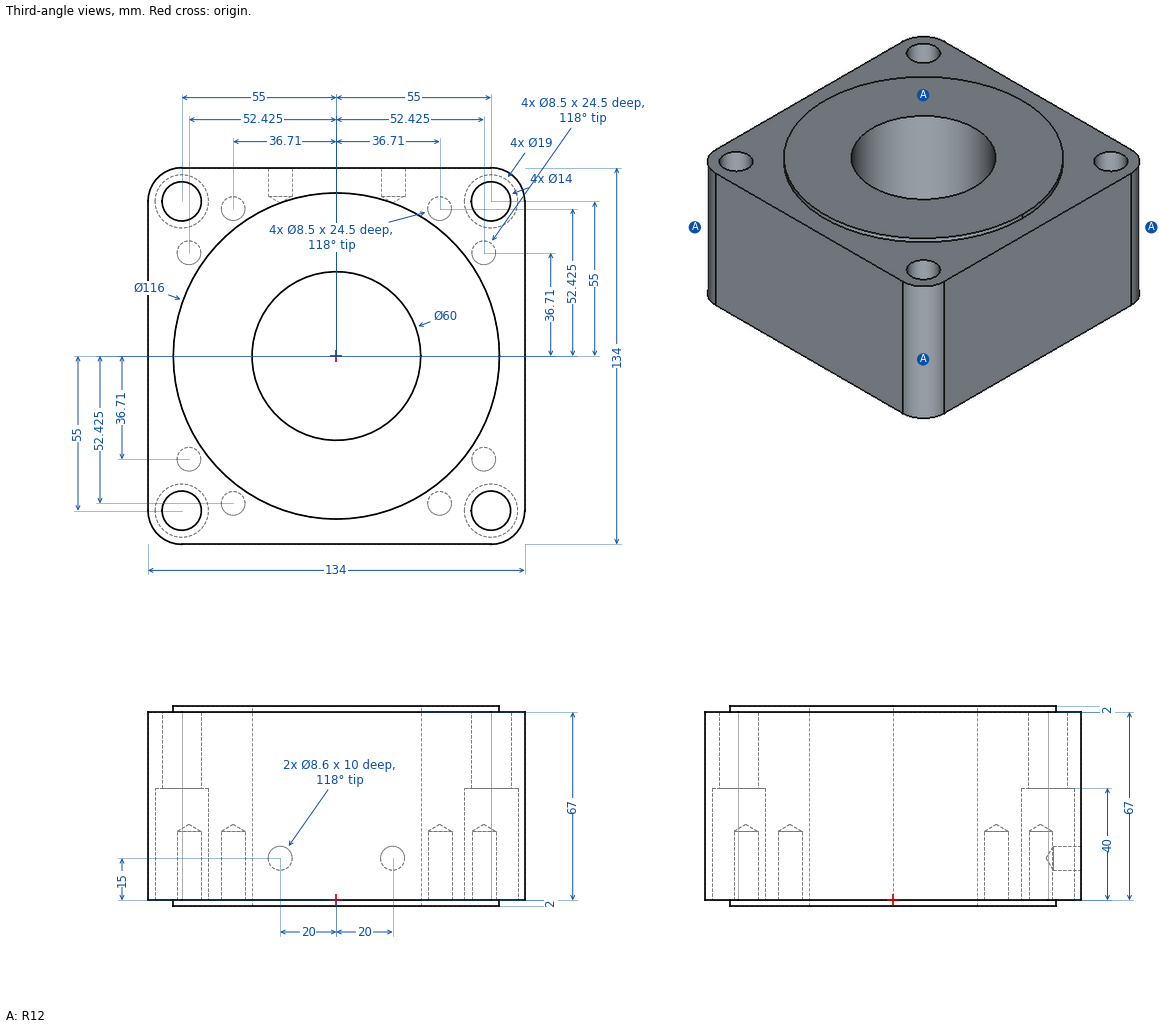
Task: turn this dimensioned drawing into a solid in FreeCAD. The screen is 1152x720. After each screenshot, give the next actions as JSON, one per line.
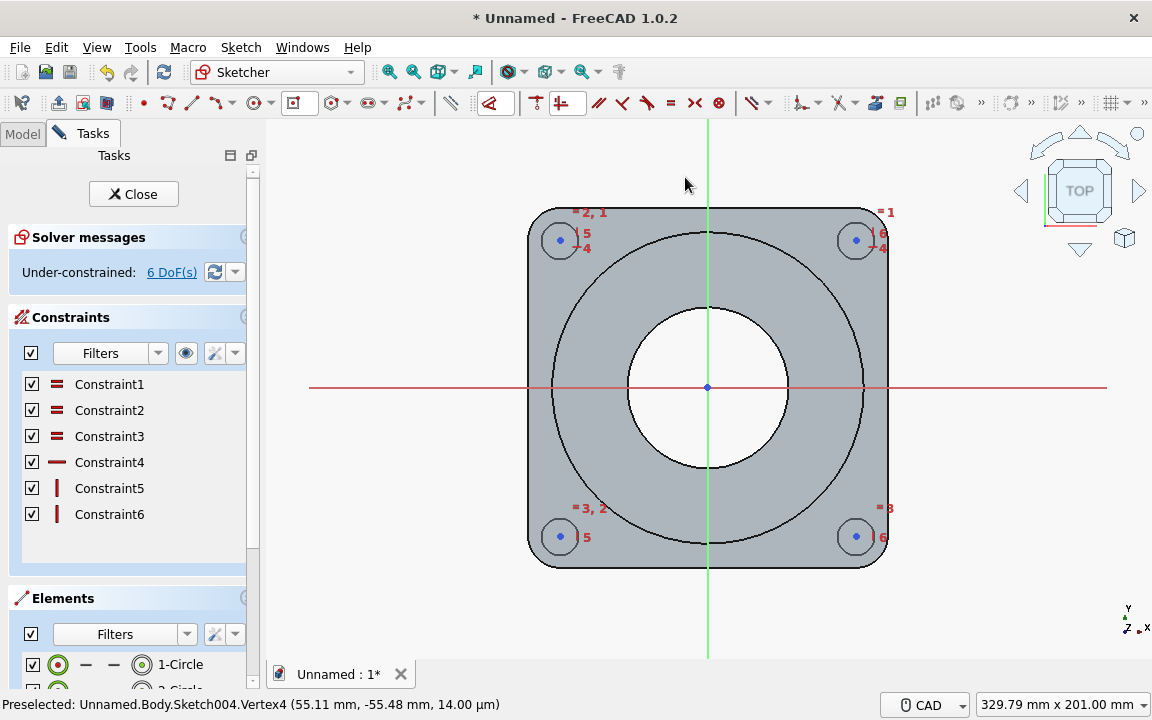
{"action": "left_click", "coordinate": [560, 537]}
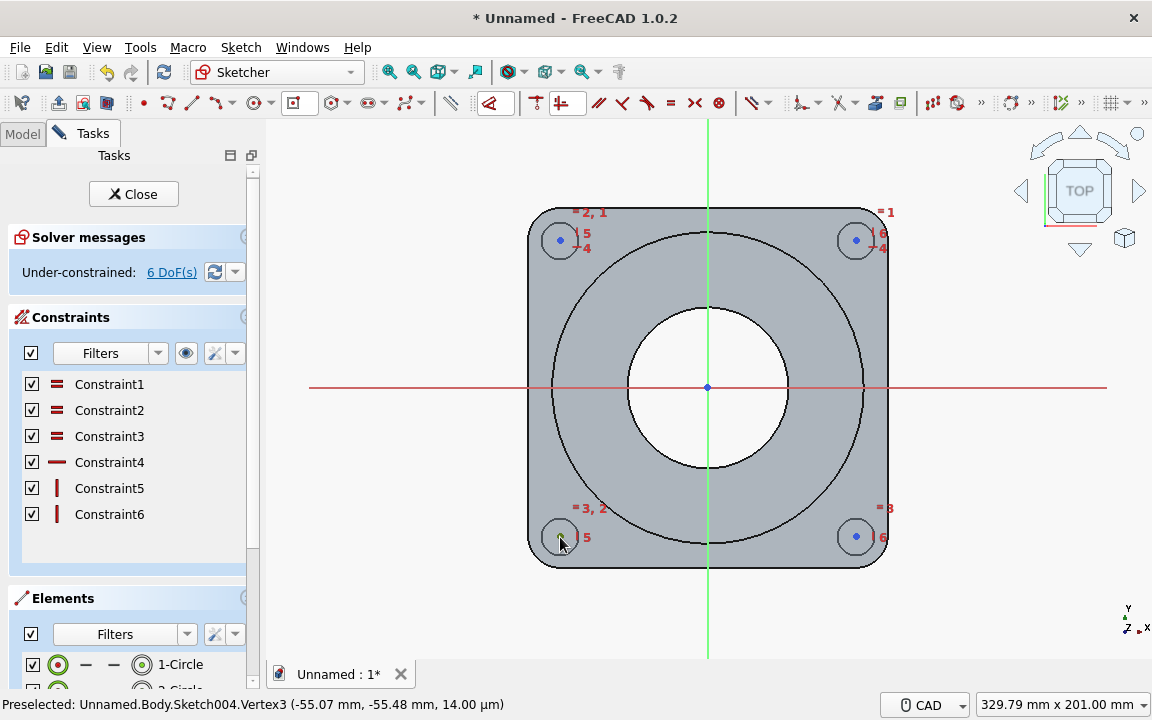
{"action": "left_click", "coordinate": [856, 537]}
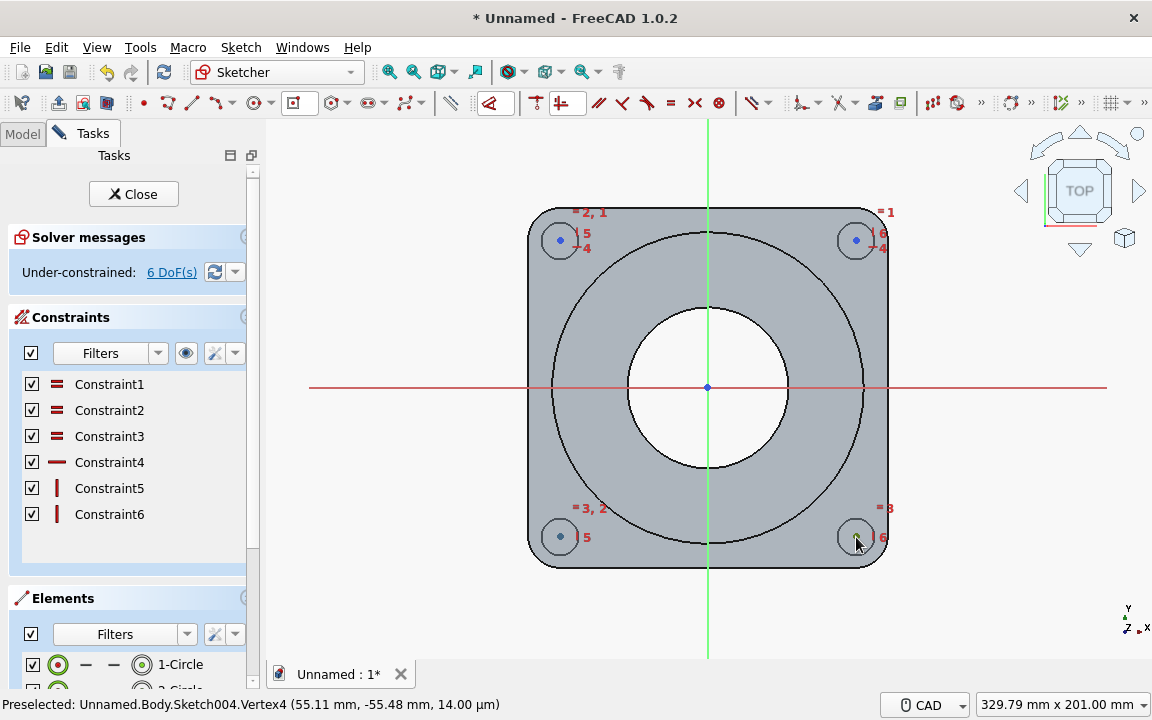
{"action": "left_click", "coordinate": [580, 104]}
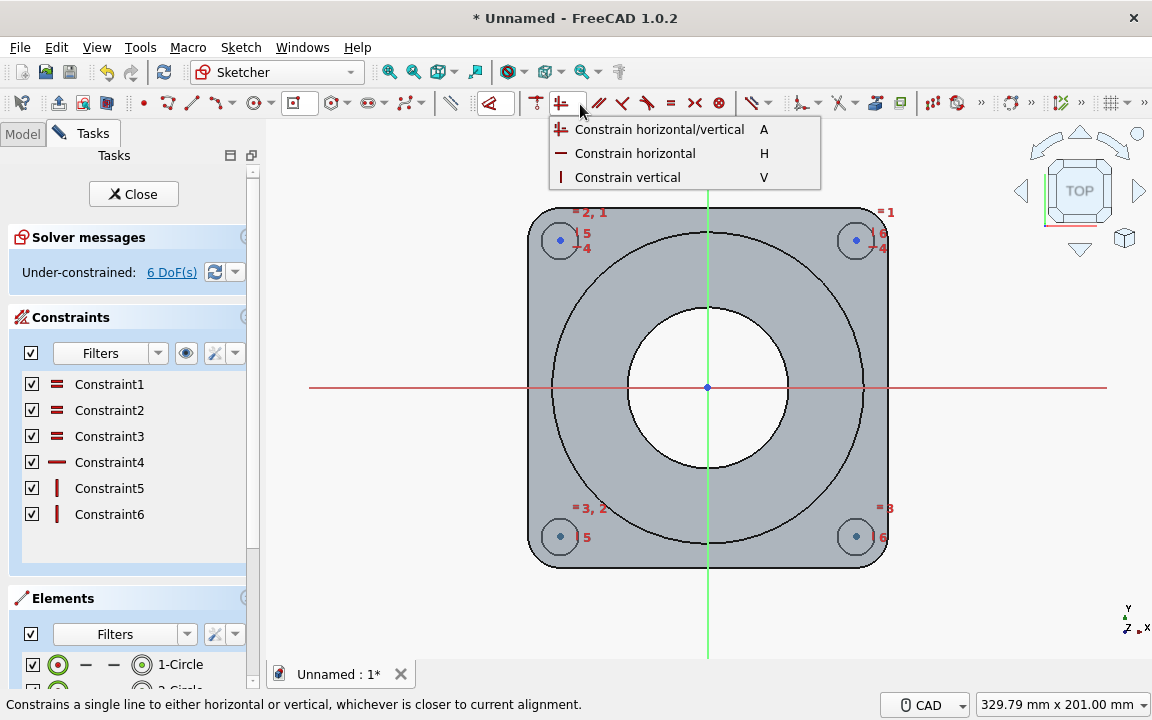
{"action": "left_click", "coordinate": [685, 153]}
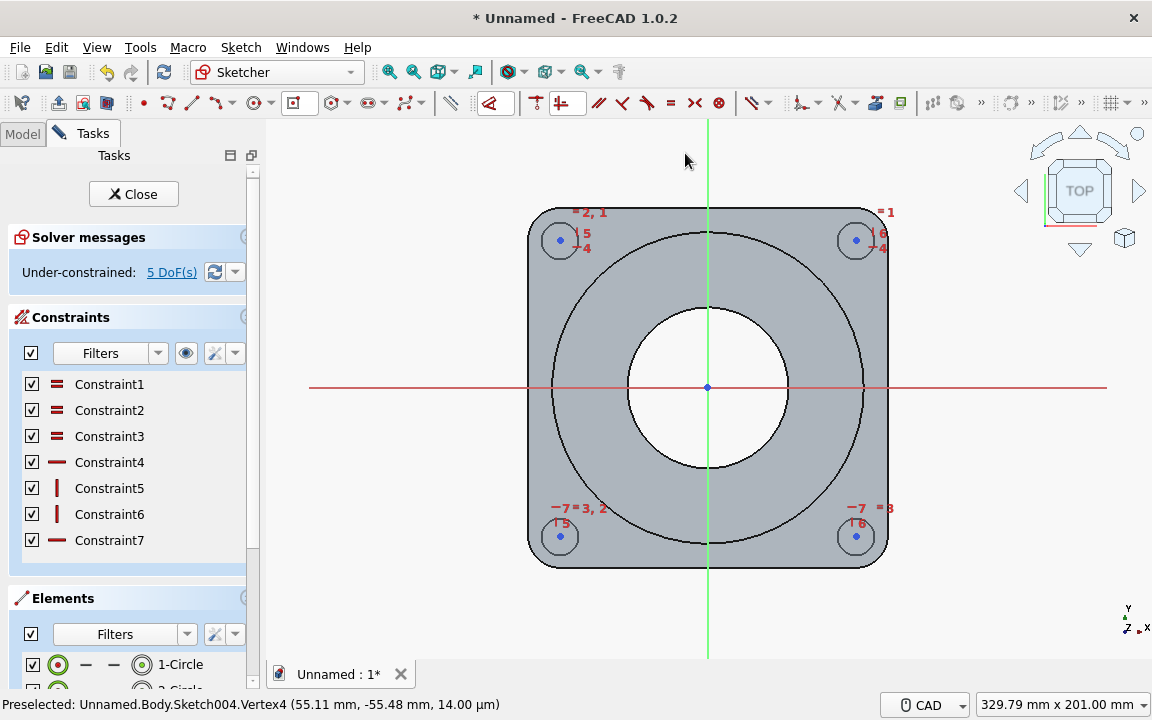
{"action": "left_click", "coordinate": [843, 228]}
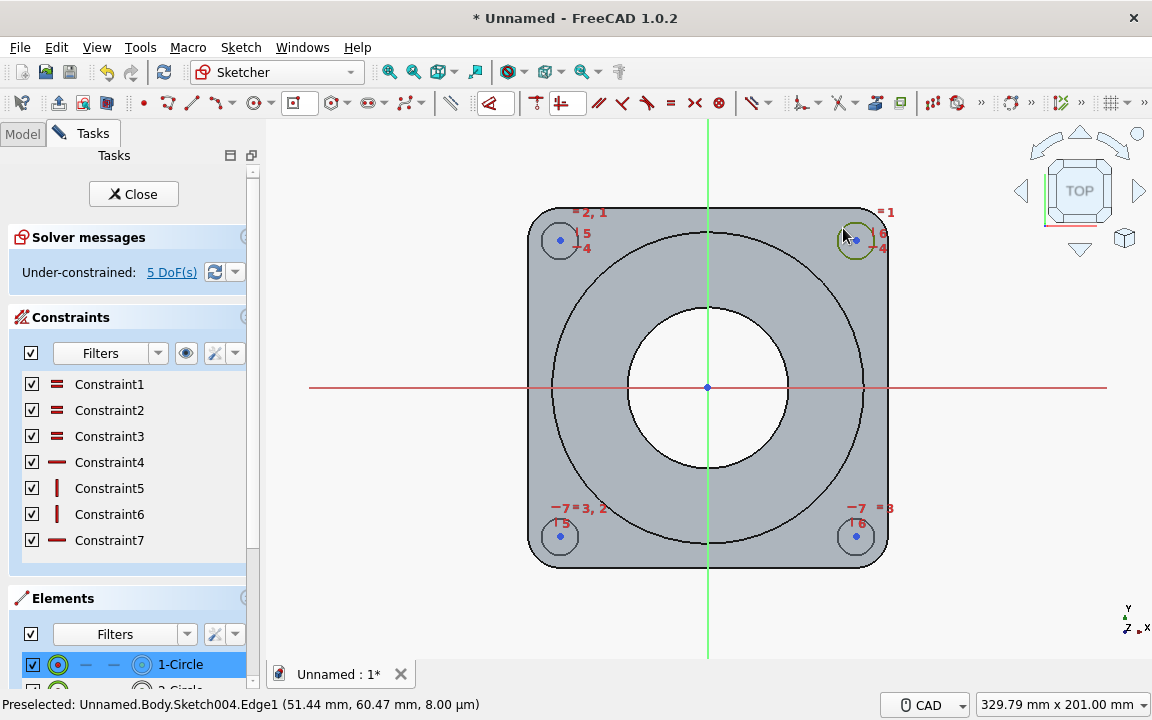
{"action": "key", "text": "k o"}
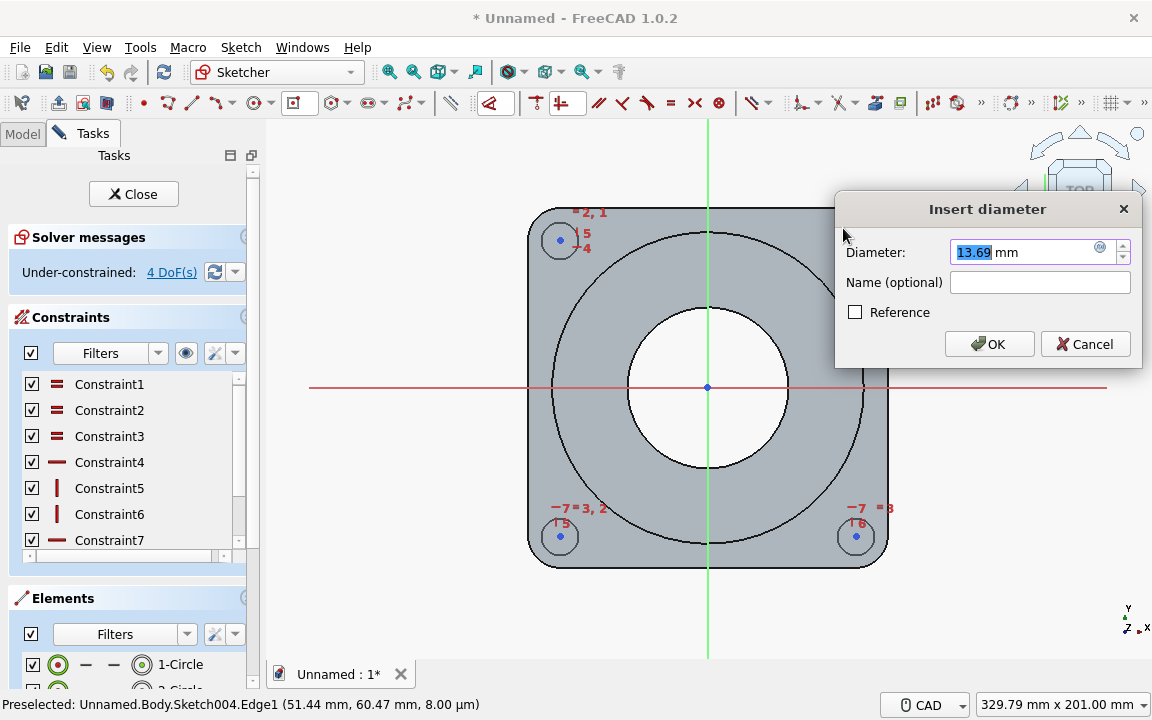
{"action": "type", "text": "14"}
{"action": "key", "text": "Return"}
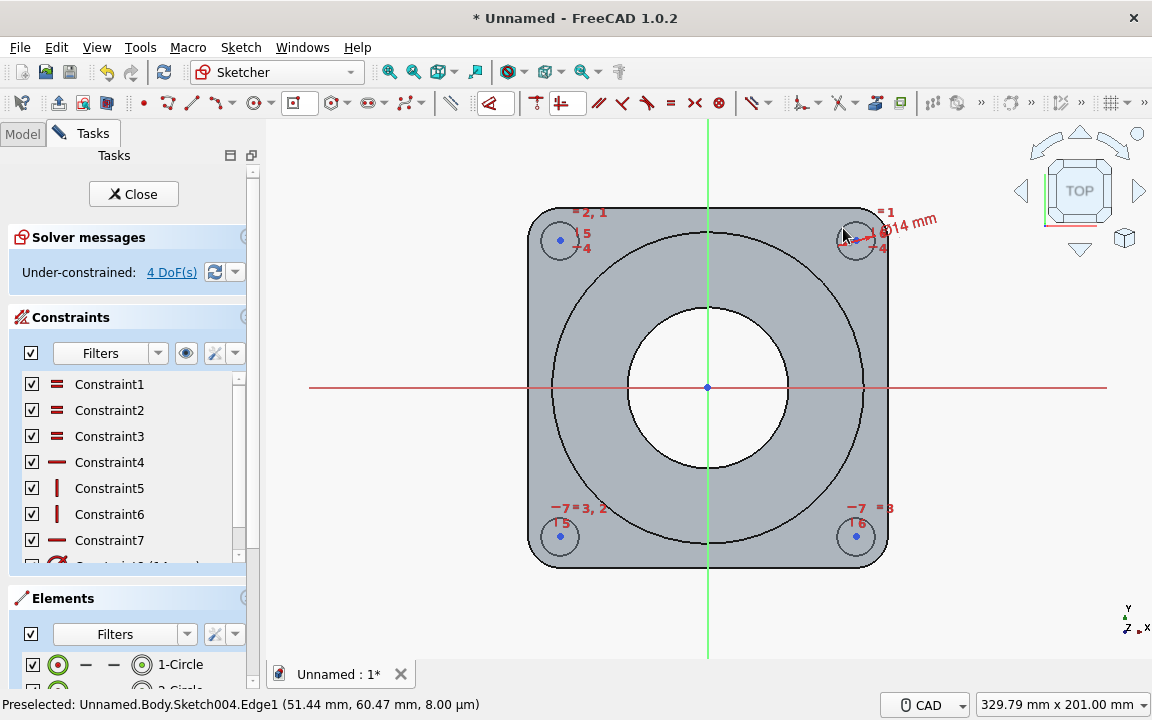
{"action": "left_click", "coordinate": [856, 241]}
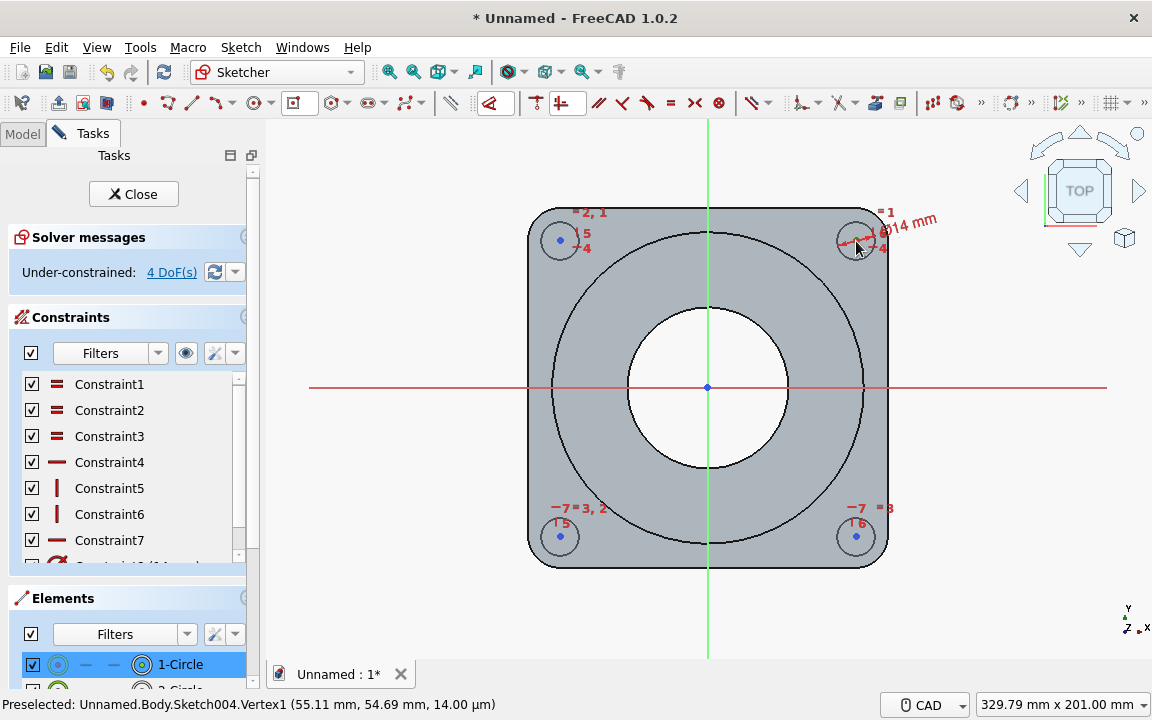
{"action": "left_click", "coordinate": [508, 104]}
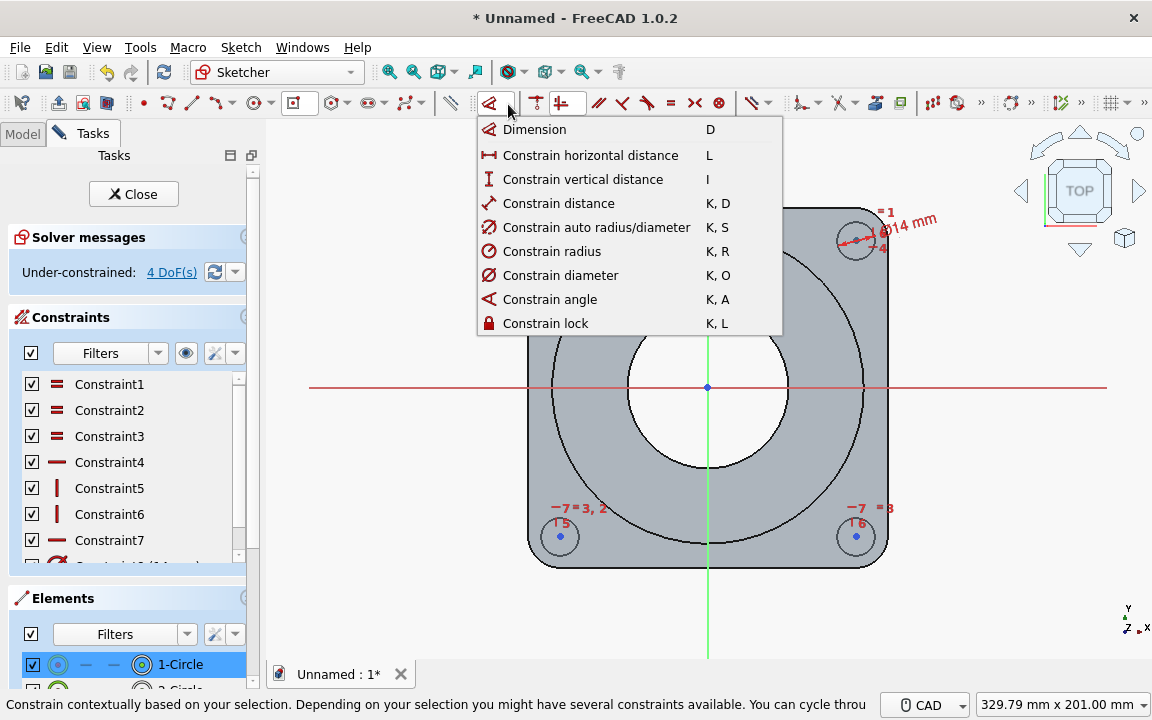
{"action": "left_click", "coordinate": [630, 155]}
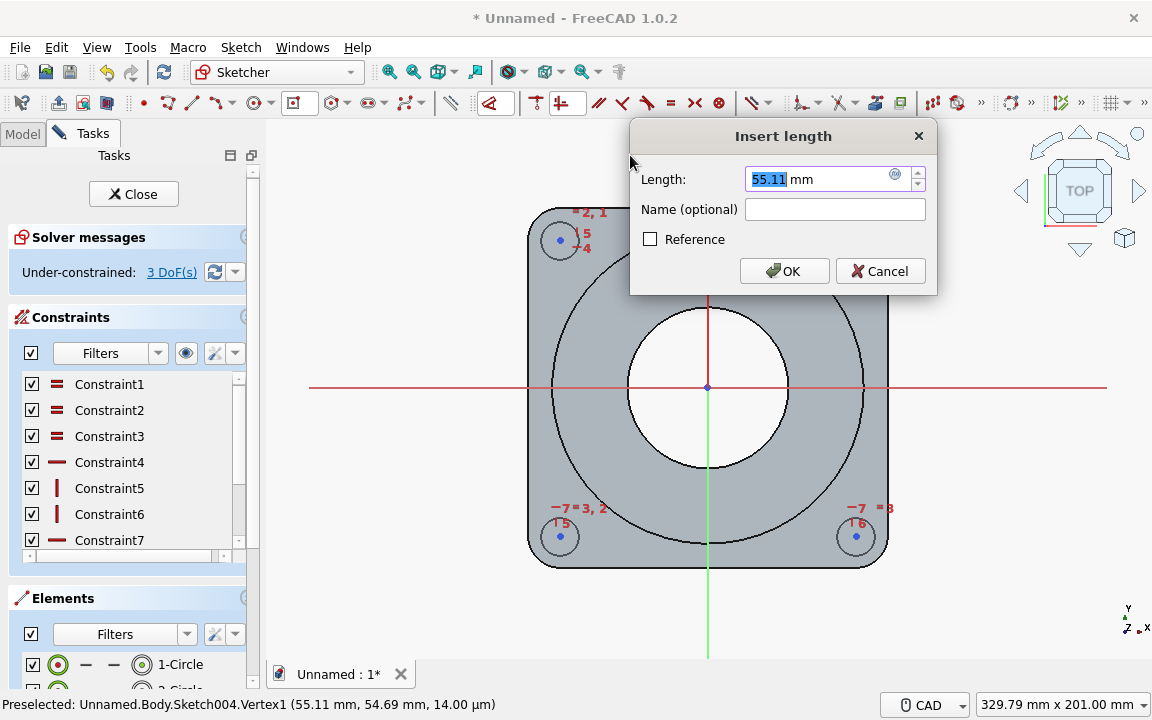
{"action": "type", "text": "55"}
{"action": "key", "text": "Return"}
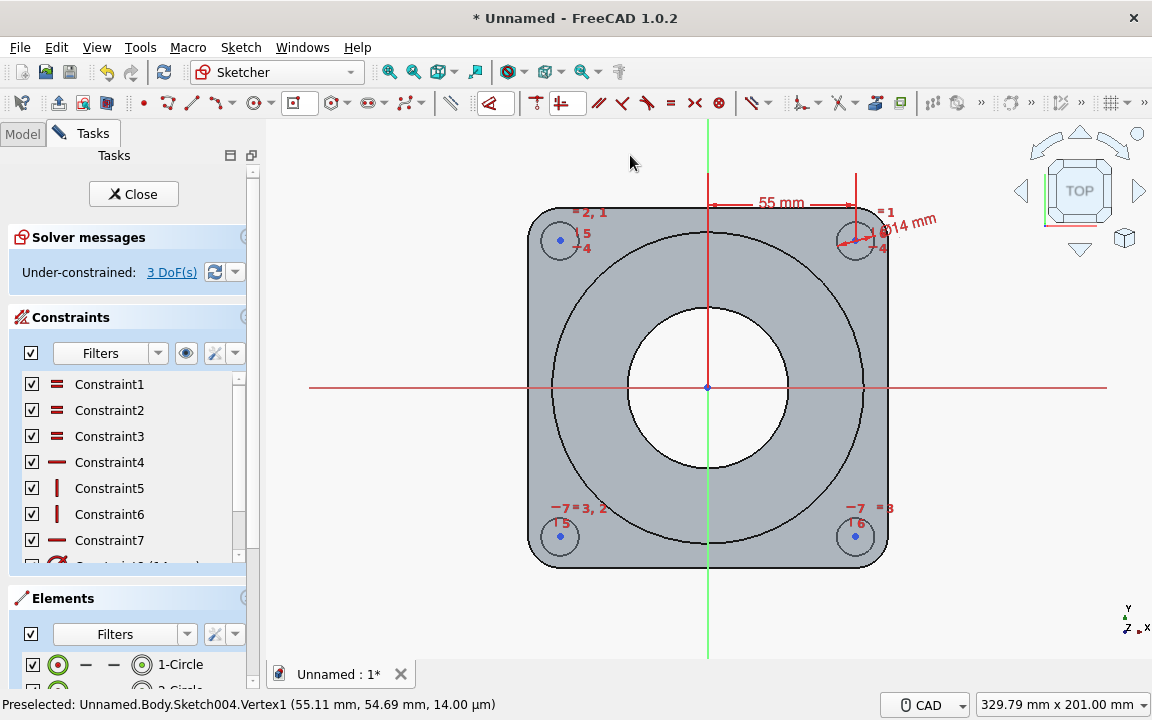
{"action": "left_click", "coordinate": [856, 241]}